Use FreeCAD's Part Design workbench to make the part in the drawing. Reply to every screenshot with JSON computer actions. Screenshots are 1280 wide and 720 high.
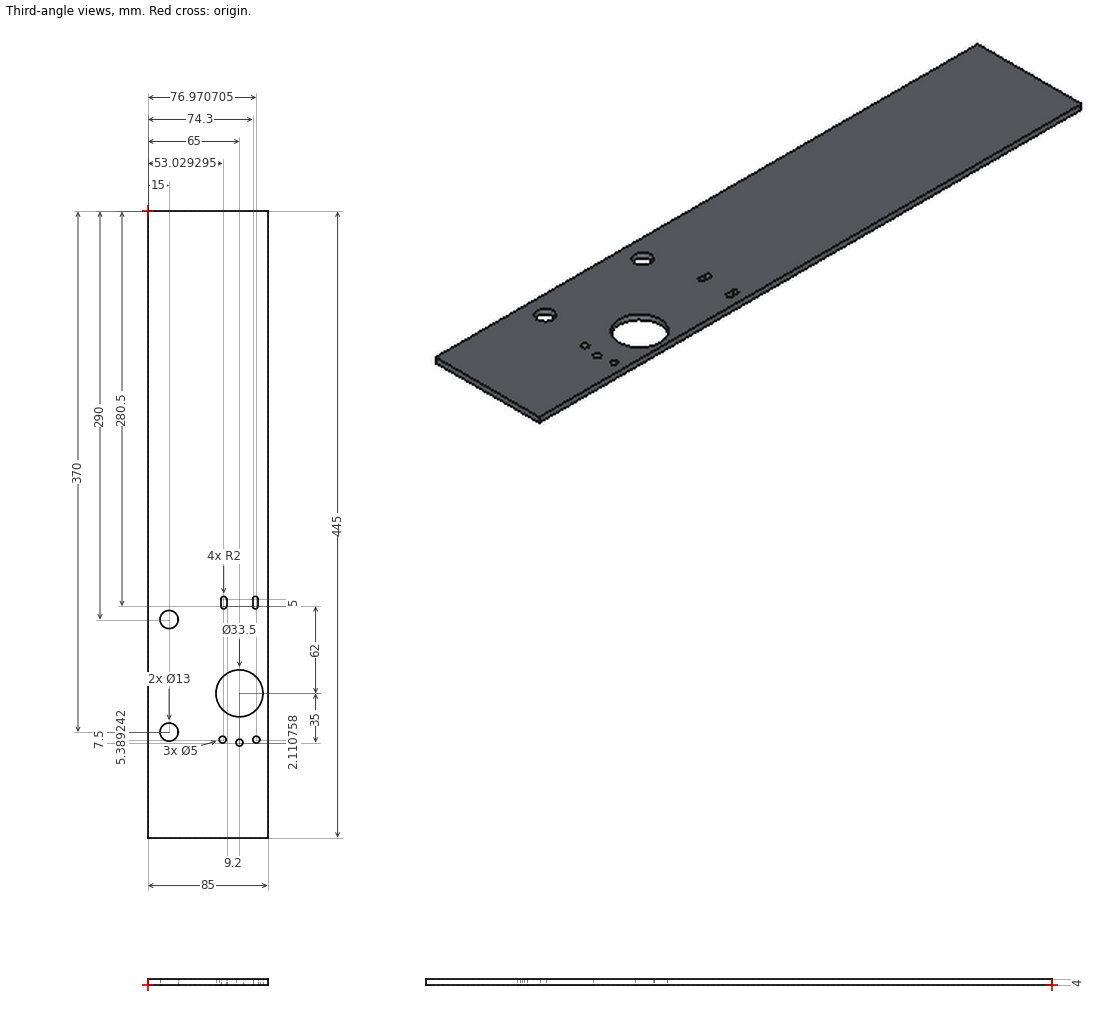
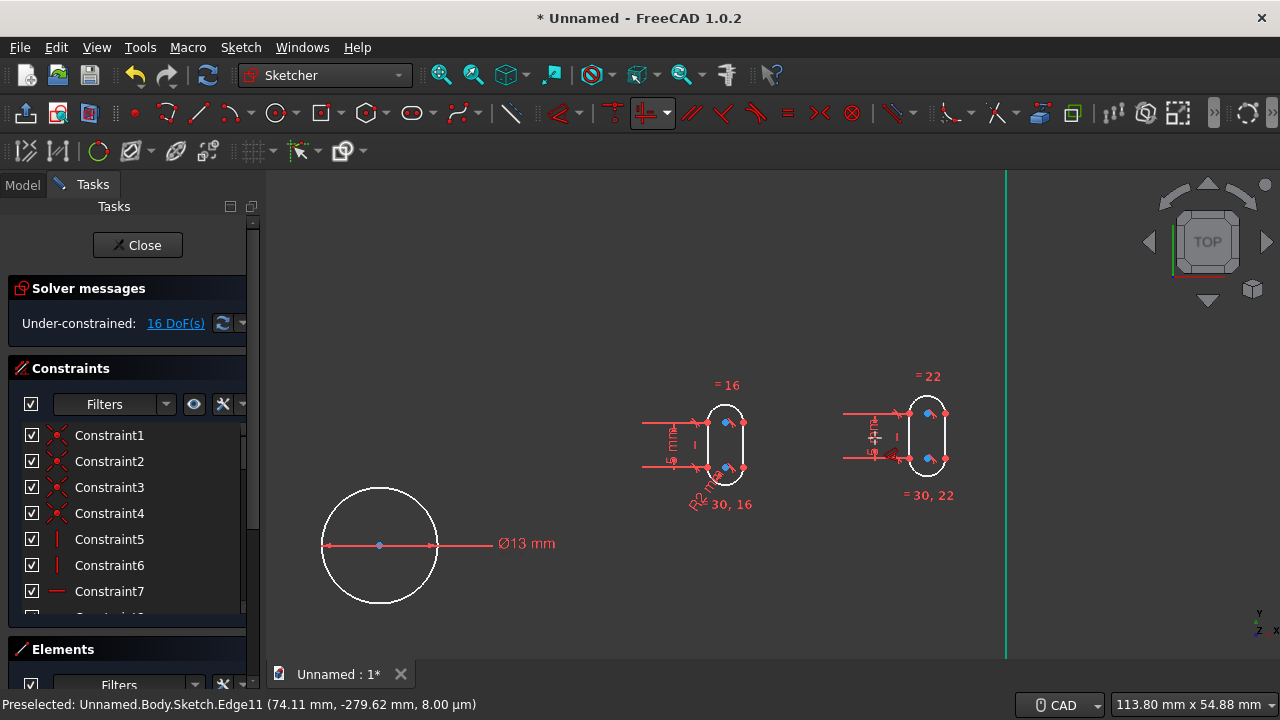
{"action": "scroll", "coordinate": [711, 453], "scroll_direction": "down", "scroll_amount": 13}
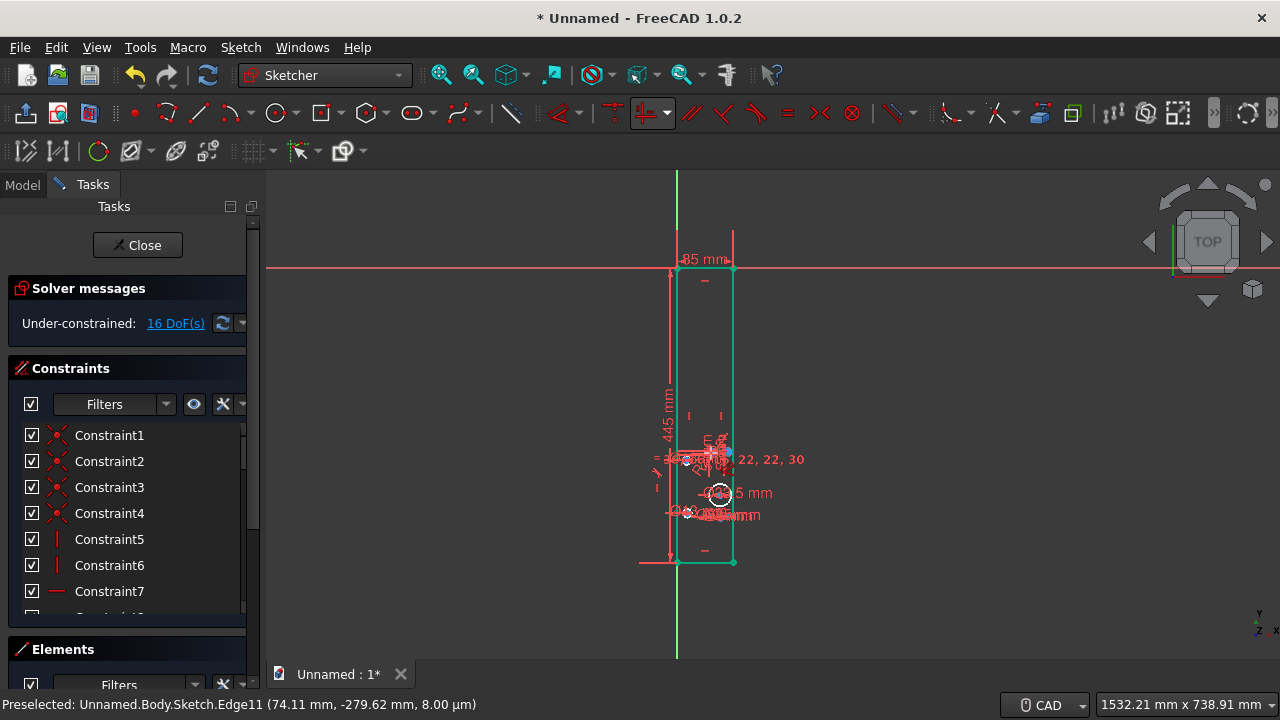
{"action": "scroll", "coordinate": [687, 513], "scroll_direction": "up", "scroll_amount": 7}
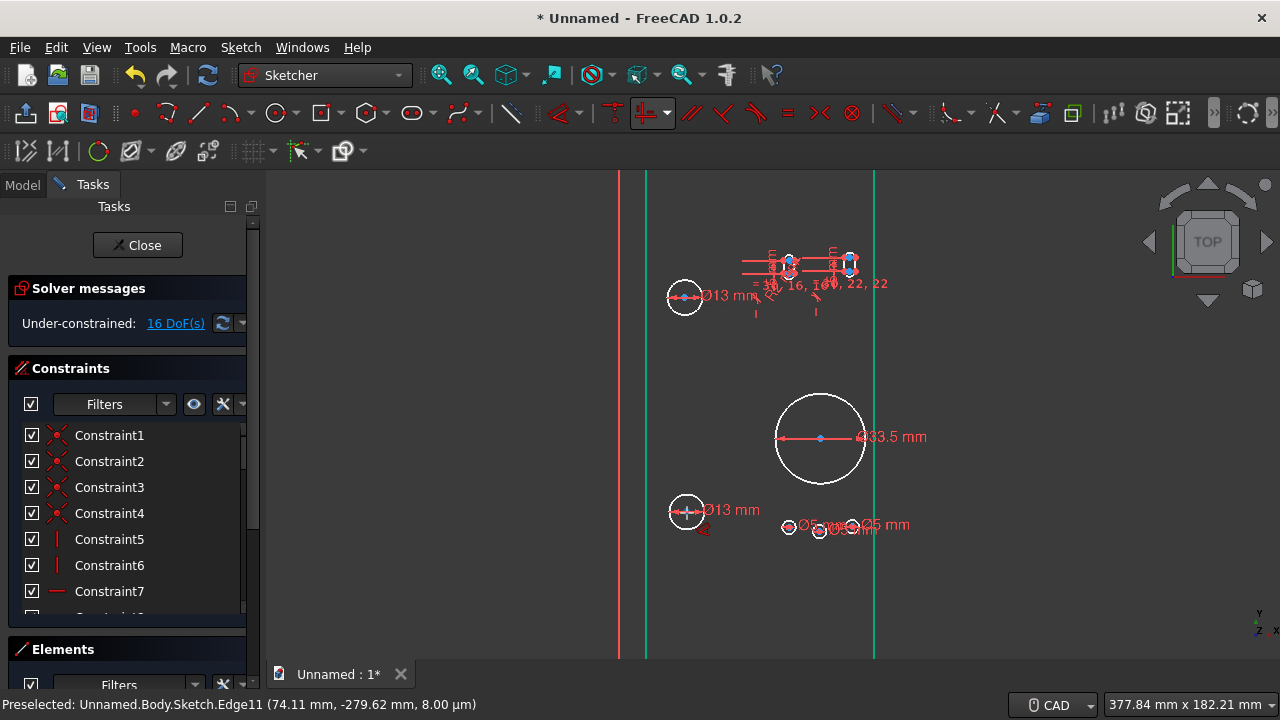
{"action": "left_click", "coordinate": [687, 512]}
{"action": "left_click", "coordinate": [666, 546]}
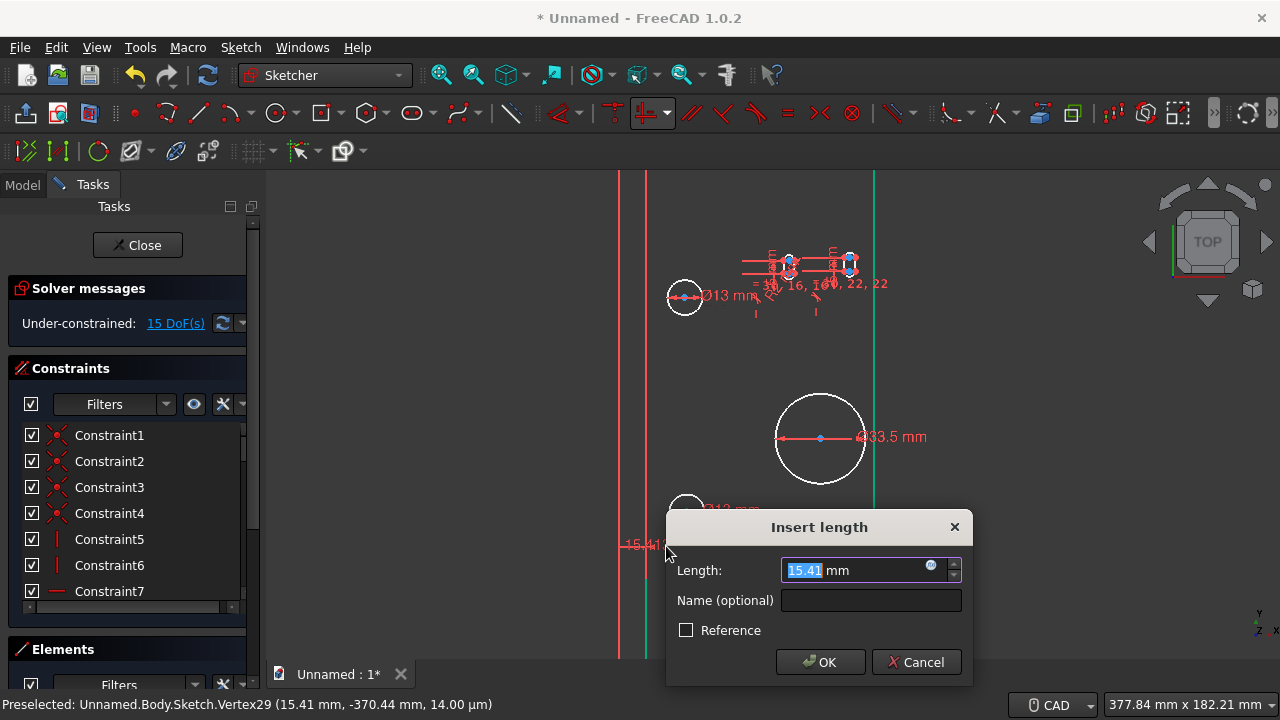
{"action": "type", "text": "15"}
{"action": "key", "text": "Return"}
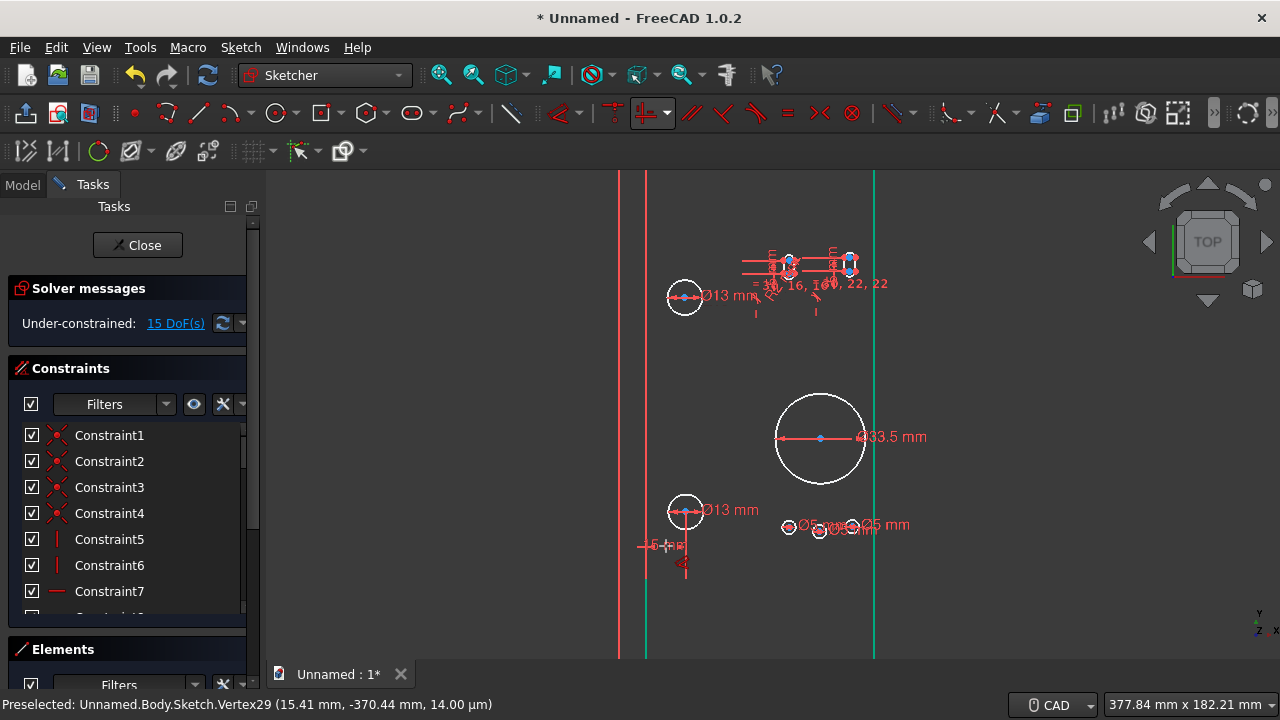
{"action": "left_click", "coordinate": [820, 532]}
{"action": "left_click", "coordinate": [773, 566]}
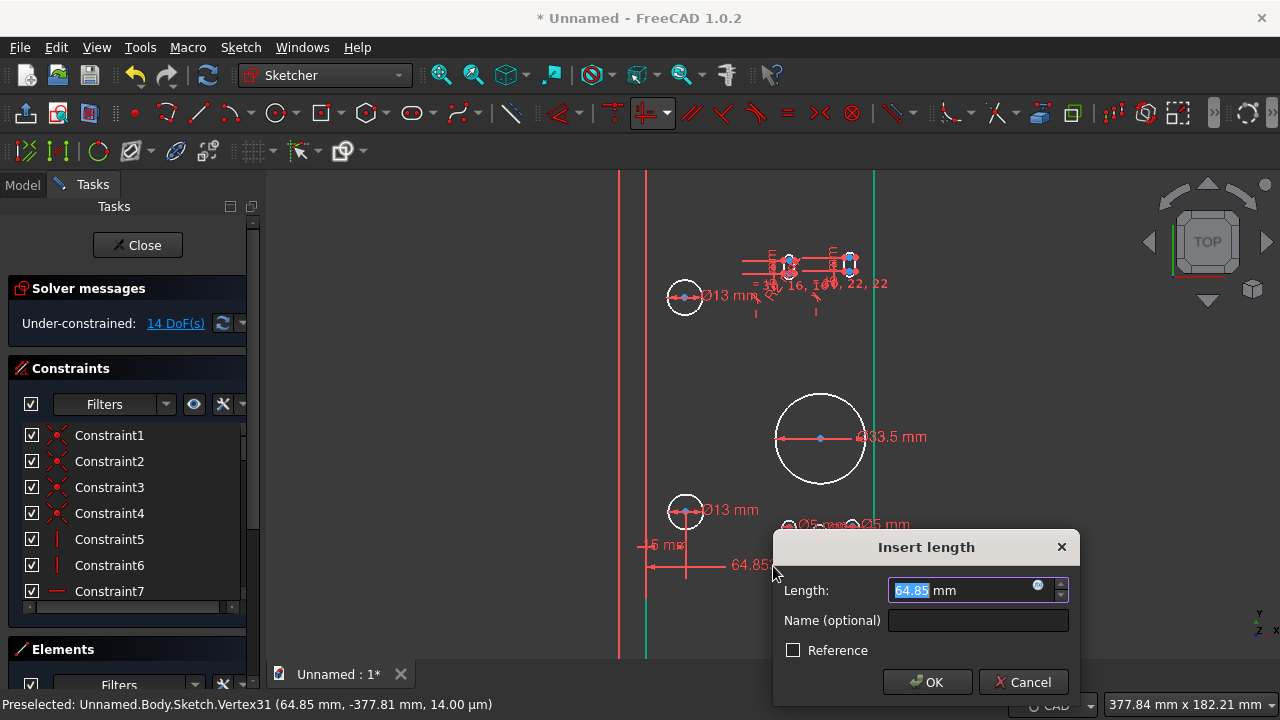
{"action": "type", "text": "65"}
{"action": "key", "text": "Return"}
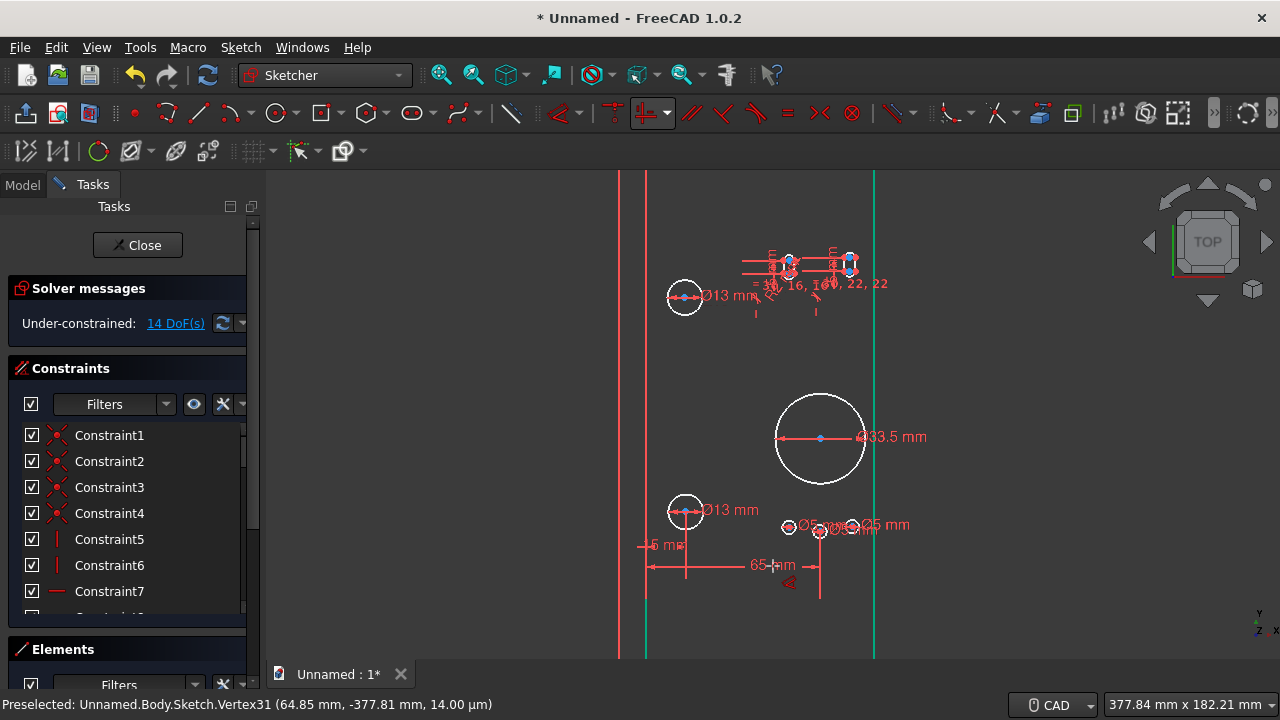
{"action": "scroll", "coordinate": [686, 513], "scroll_direction": "down", "scroll_amount": 7}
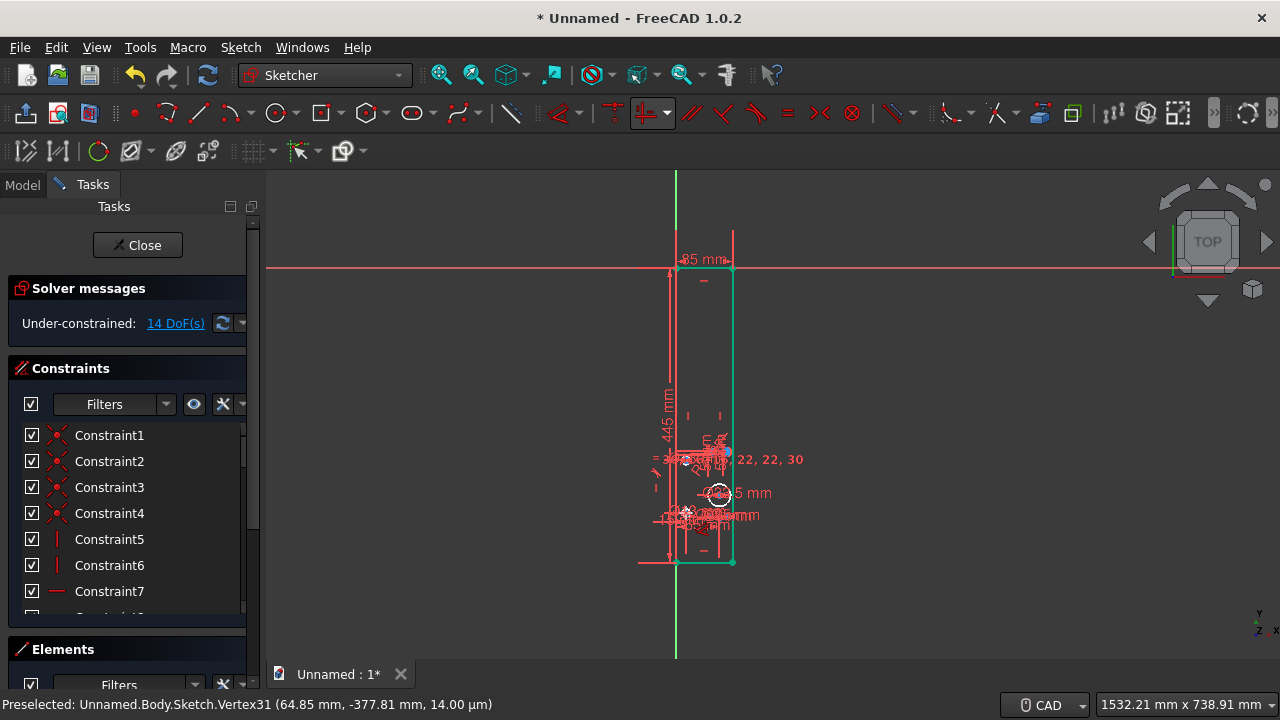
{"action": "left_click", "coordinate": [719, 495]}
{"action": "left_click", "coordinate": [698, 234]}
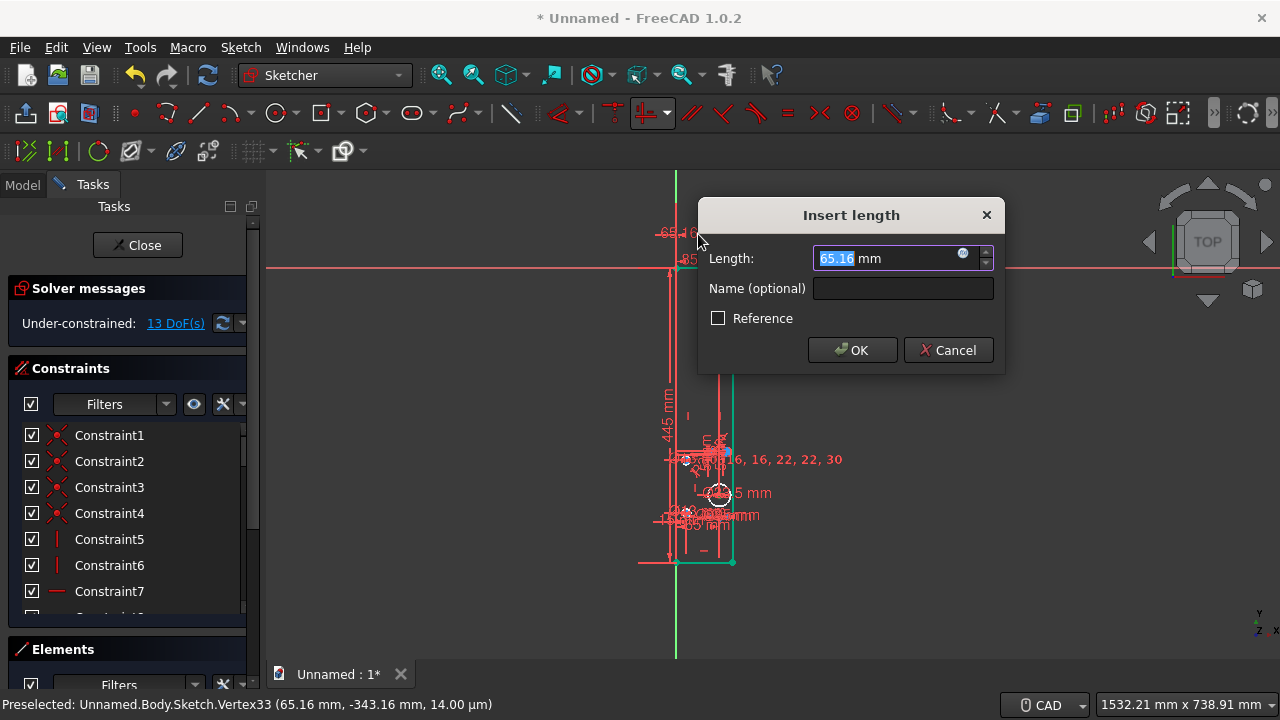
{"action": "type", "text": "65"}
{"action": "key", "text": "Return"}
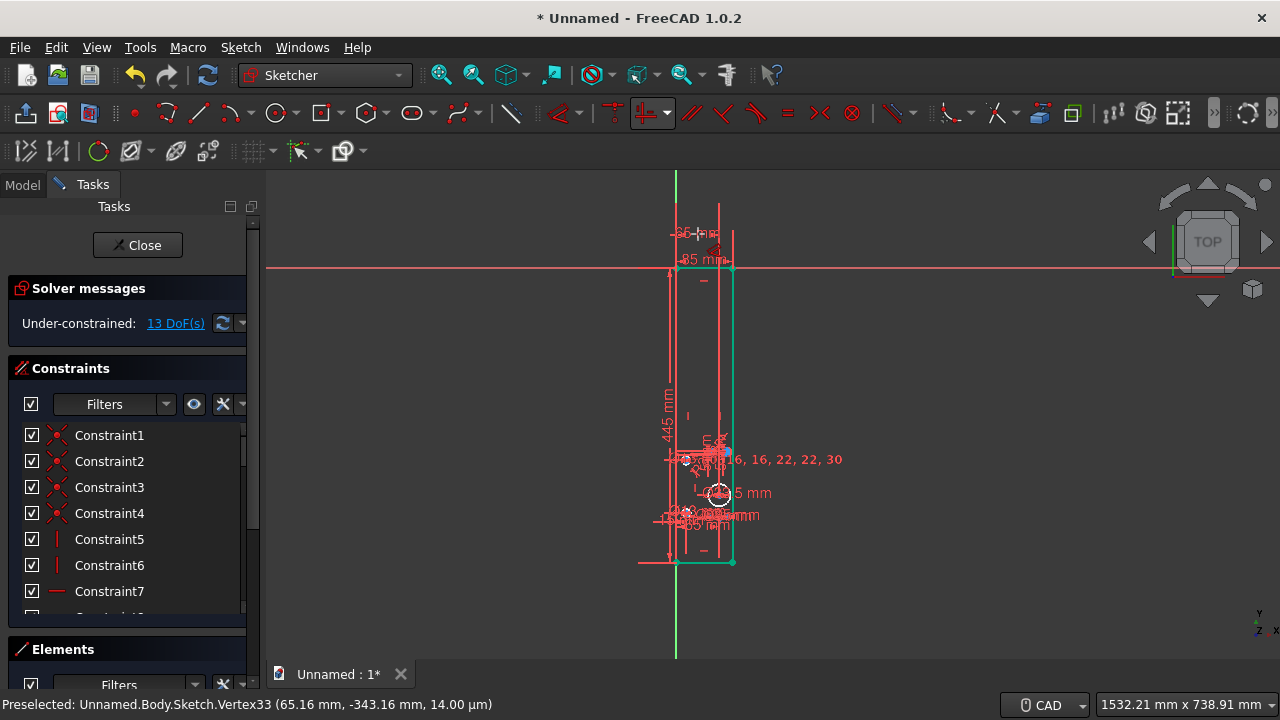
{"action": "scroll", "coordinate": [686, 460], "scroll_direction": "up", "scroll_amount": 7}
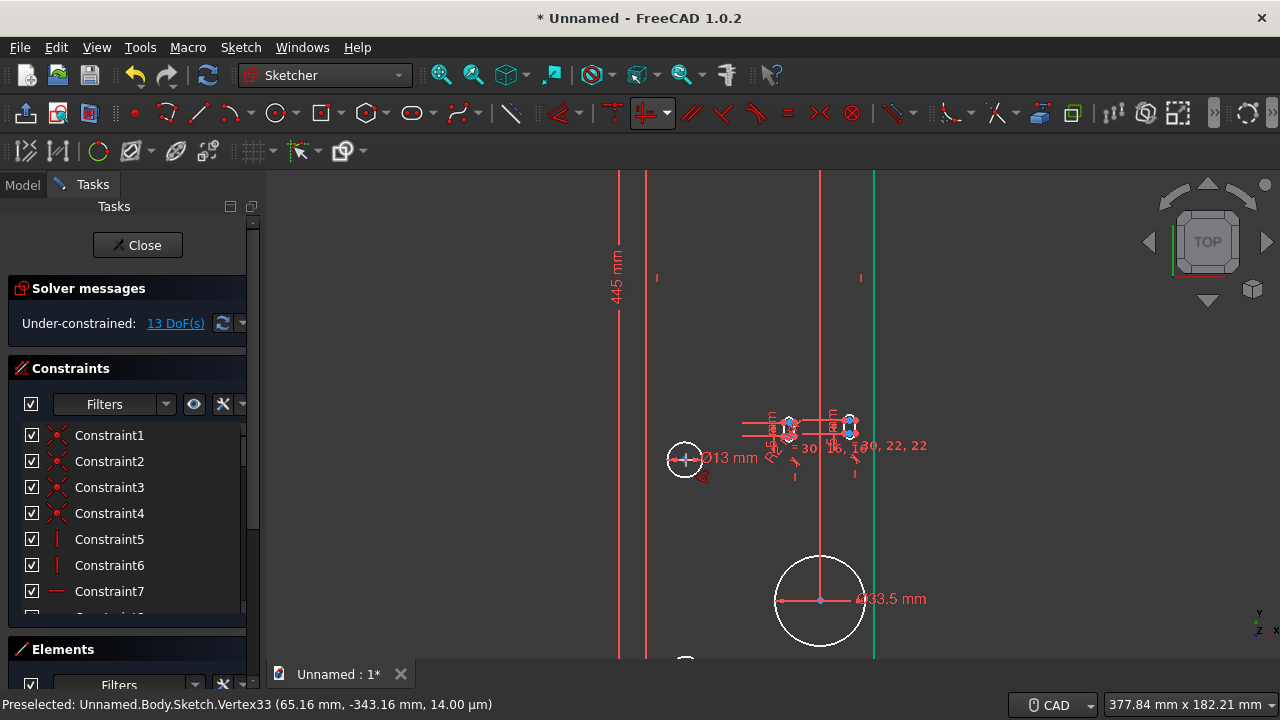
{"action": "left_click", "coordinate": [685, 460]}
{"action": "left_click", "coordinate": [665, 494]}